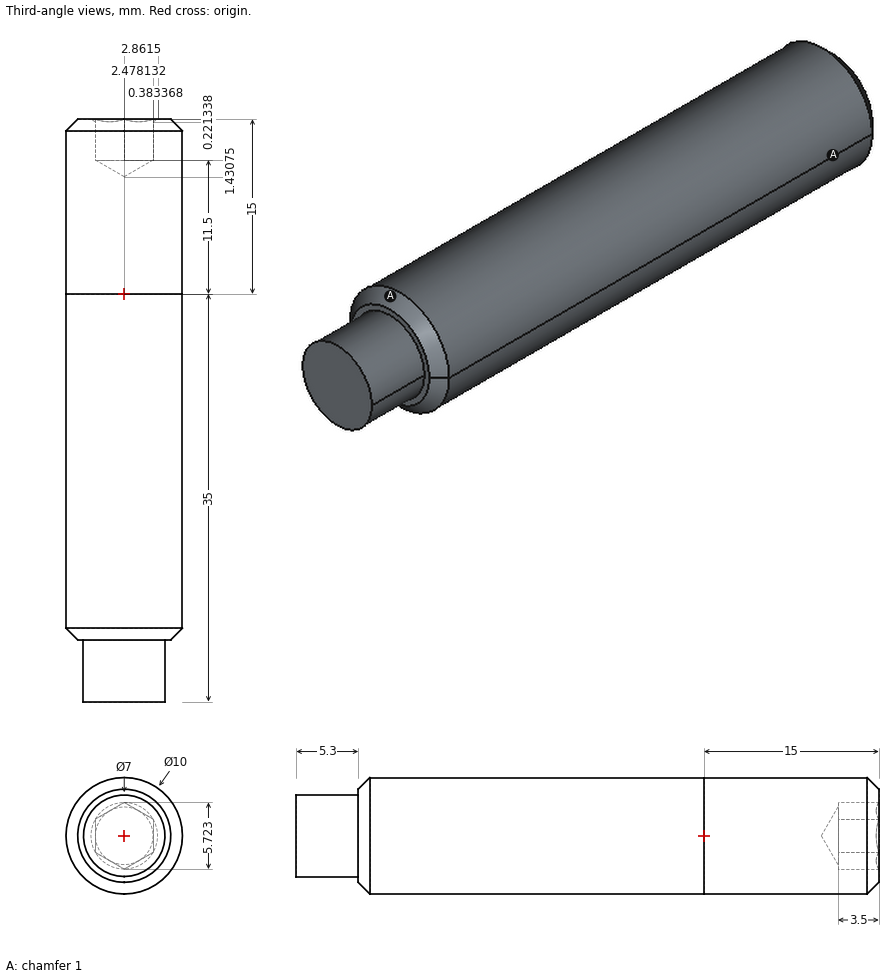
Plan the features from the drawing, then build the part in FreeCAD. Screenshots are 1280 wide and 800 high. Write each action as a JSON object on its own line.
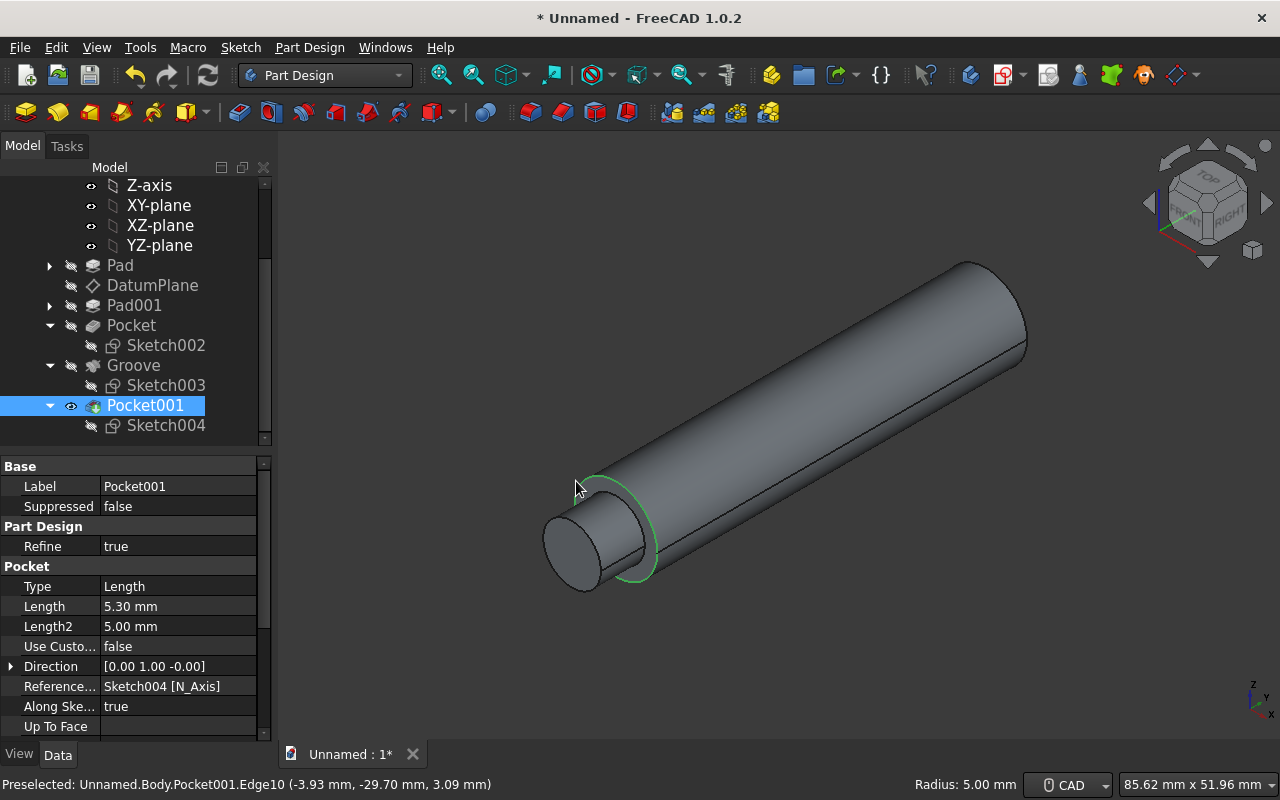
{"action": "key", "text": "2"}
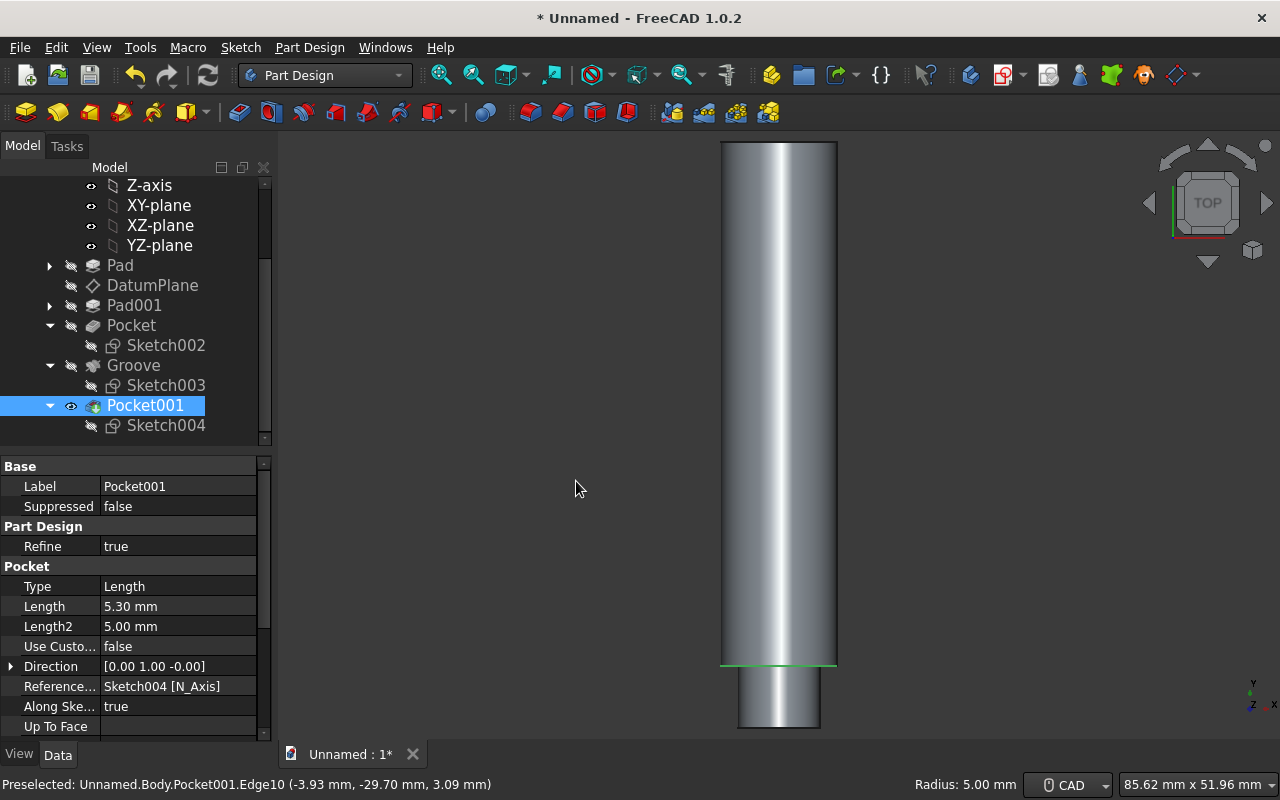
{"action": "key", "text": "0"}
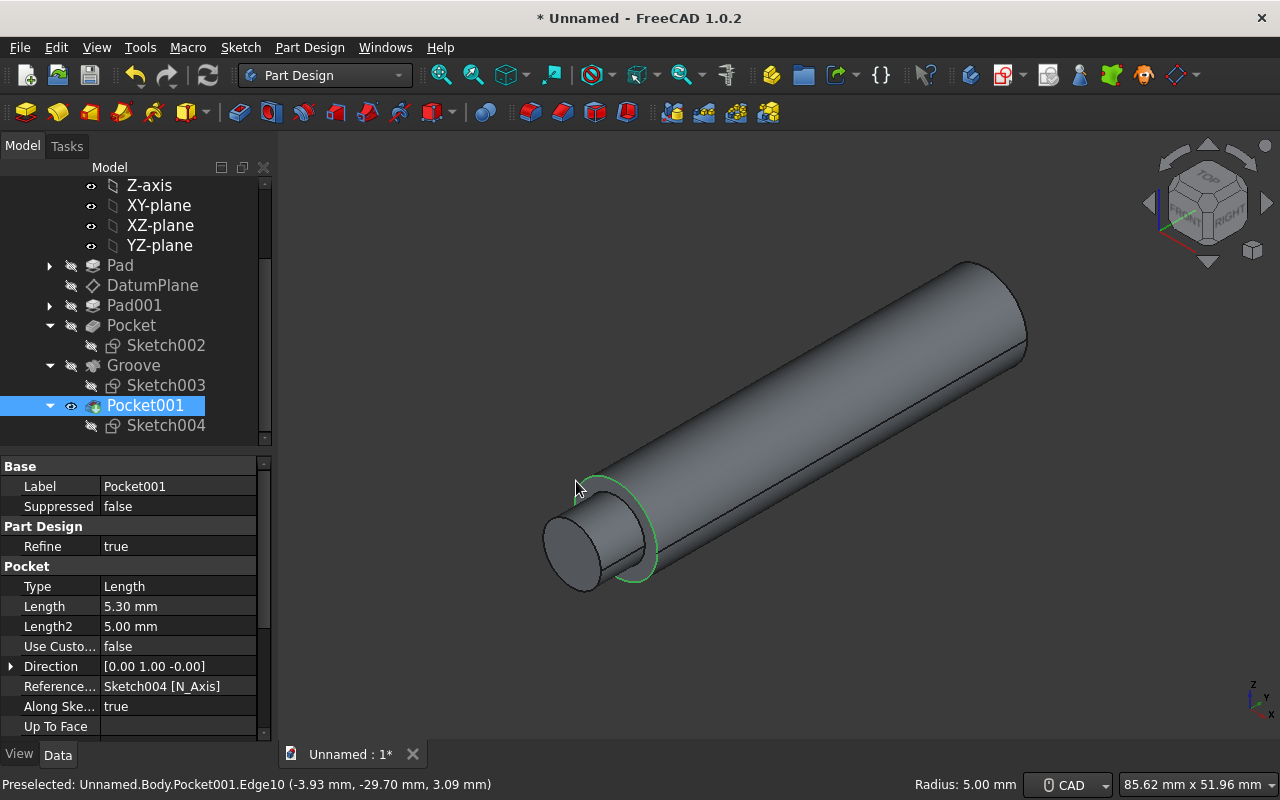
{"action": "key", "text": "1"}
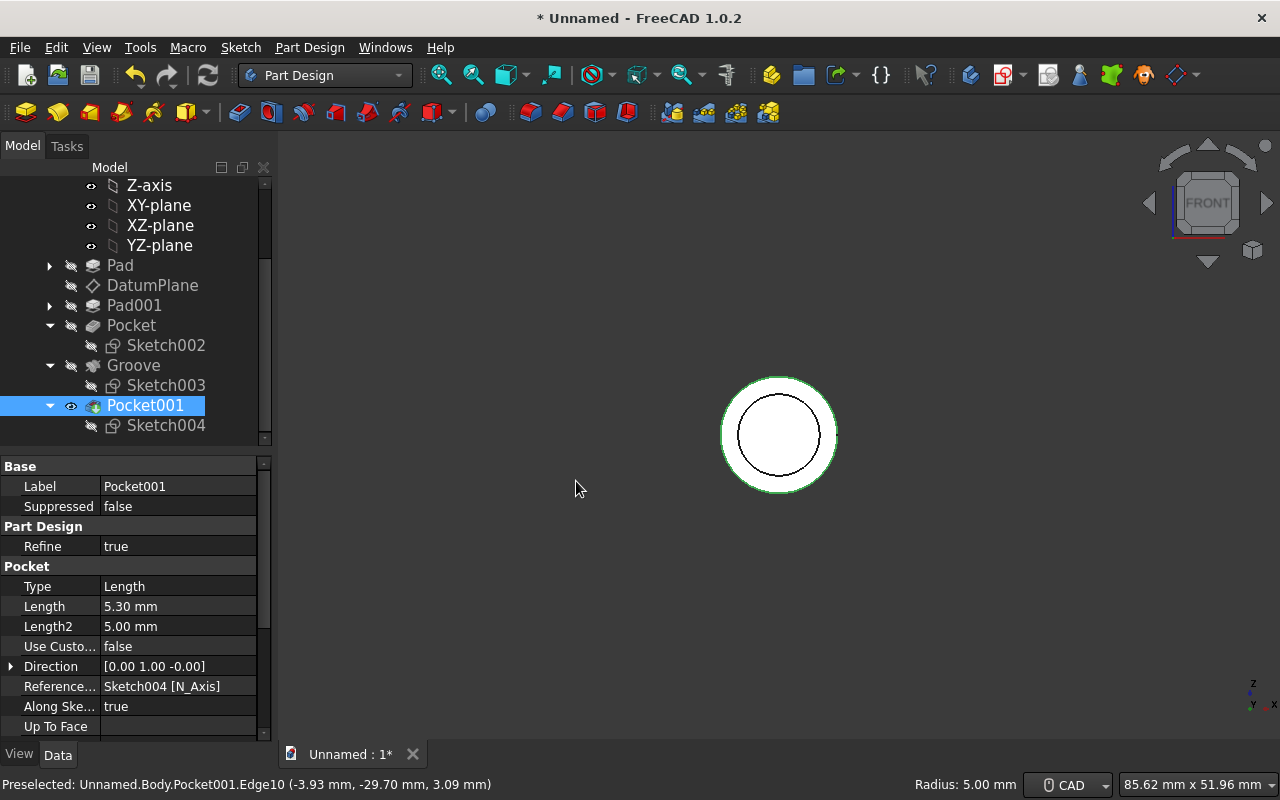
{"action": "left_click", "coordinate": [442, 76]}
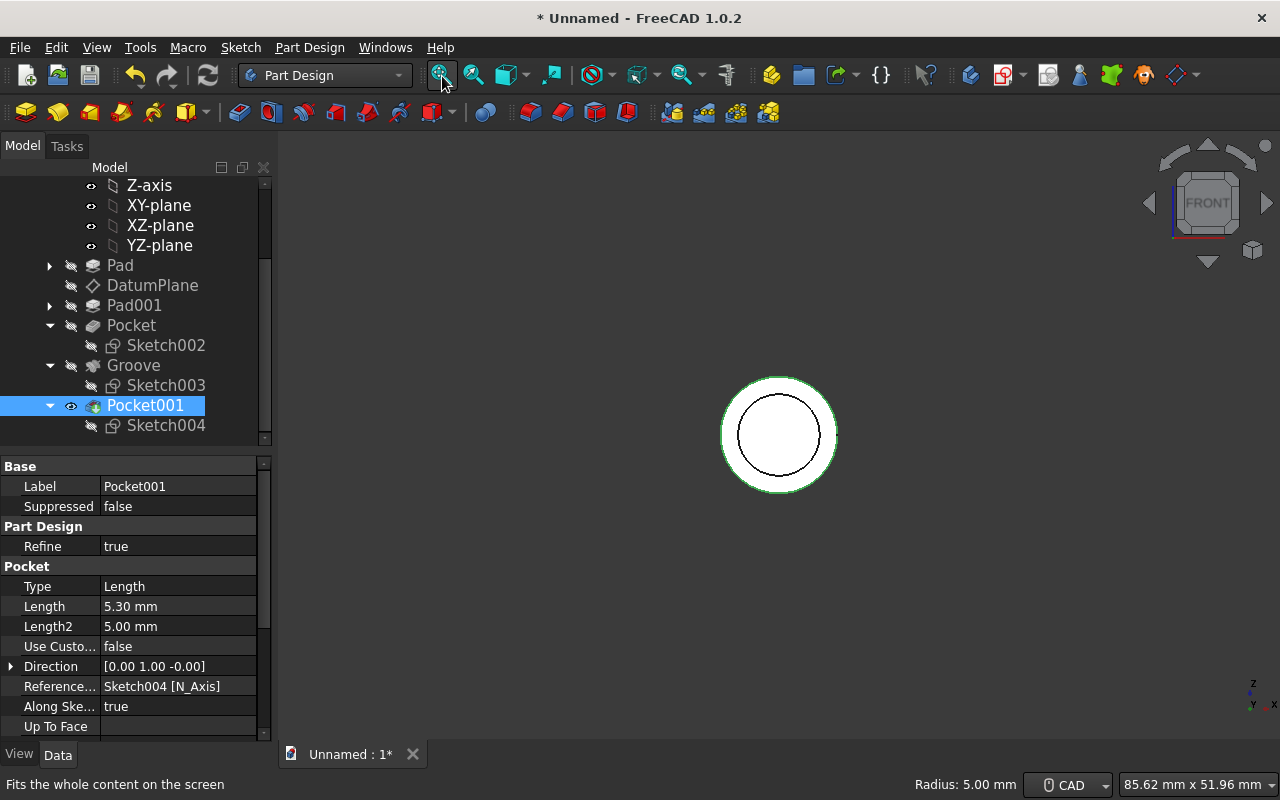
{"action": "key", "text": "3"}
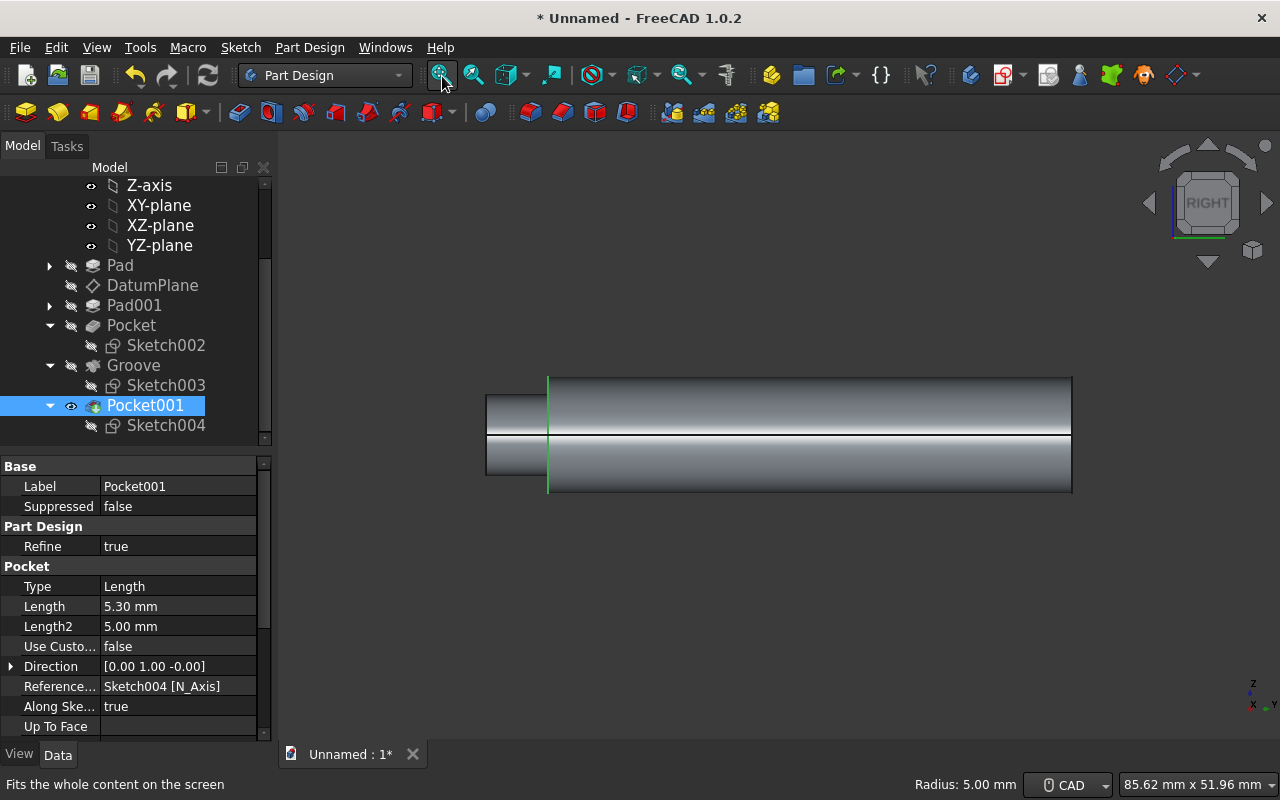
{"action": "left_click", "coordinate": [1072, 400], "text": "ctrl"}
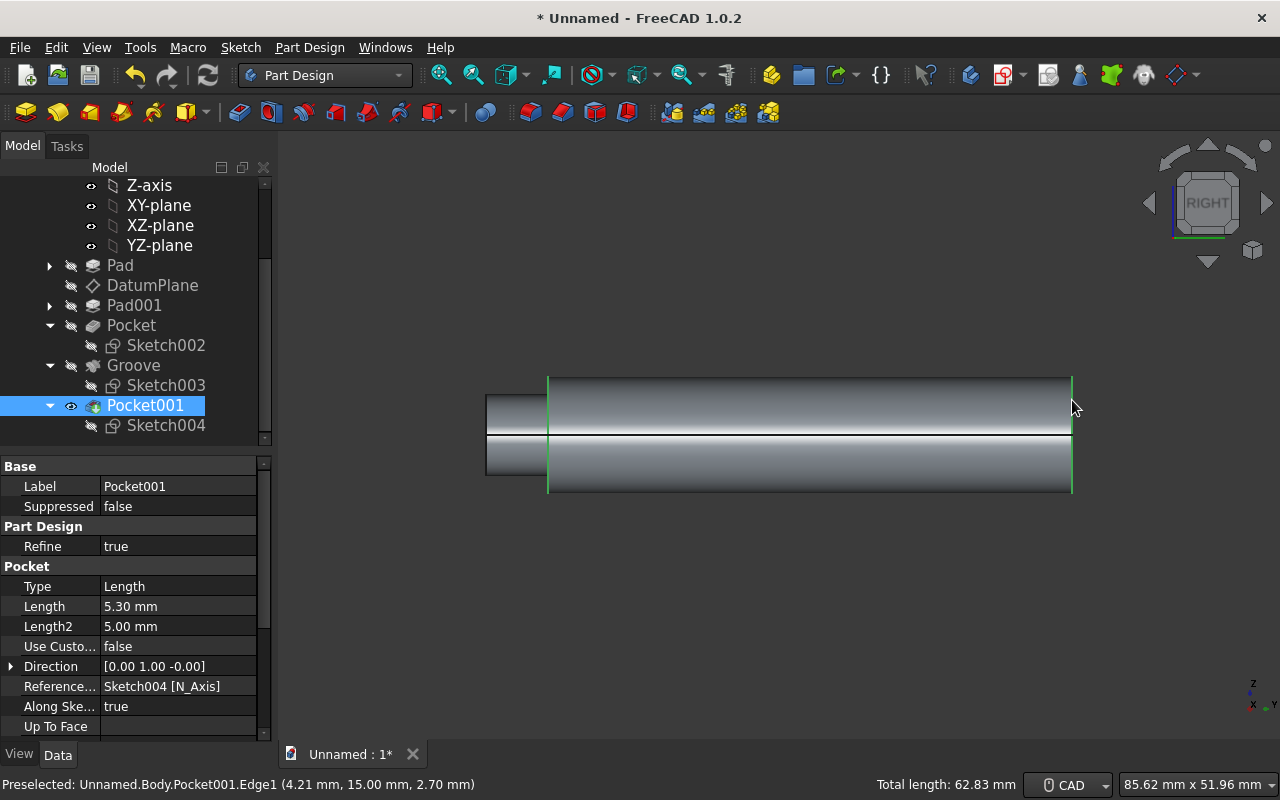
{"action": "left_click", "coordinate": [564, 112]}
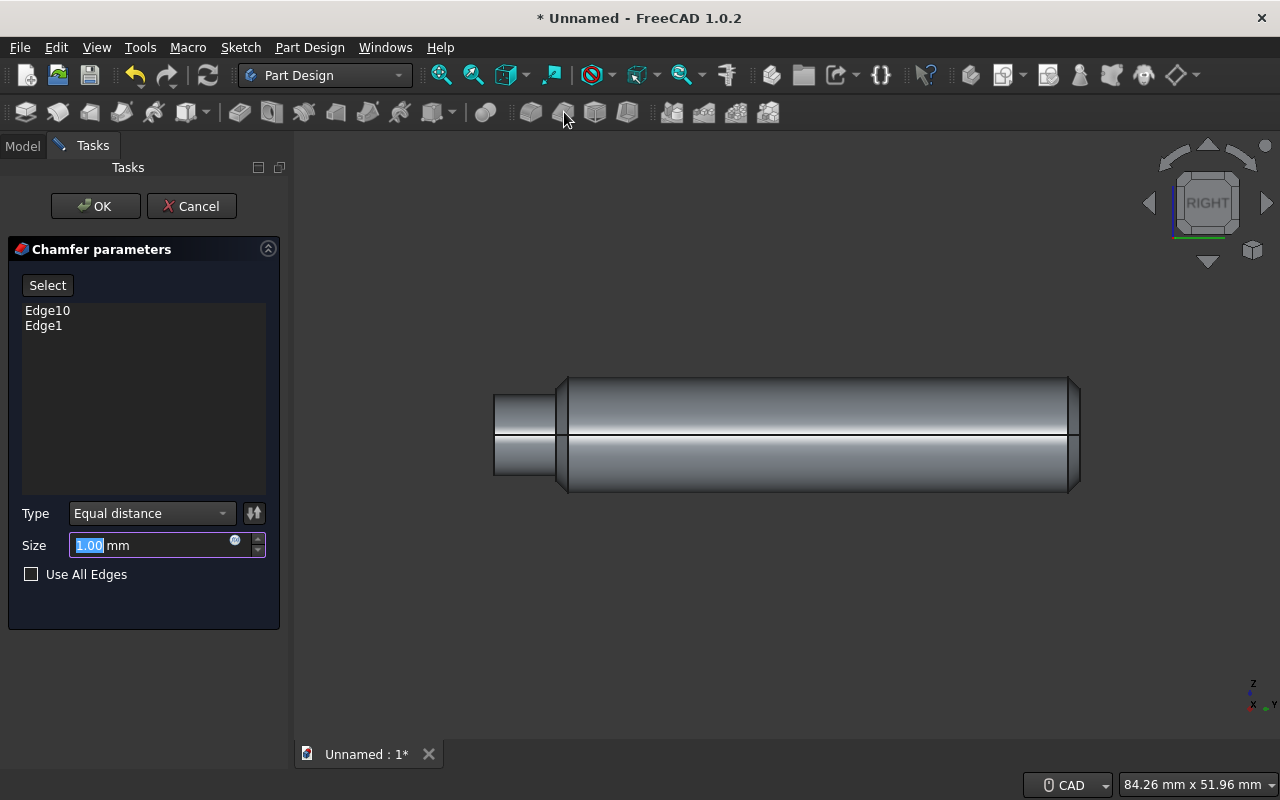
{"action": "type", "text": "1"}
{"action": "key", "text": "Tab"}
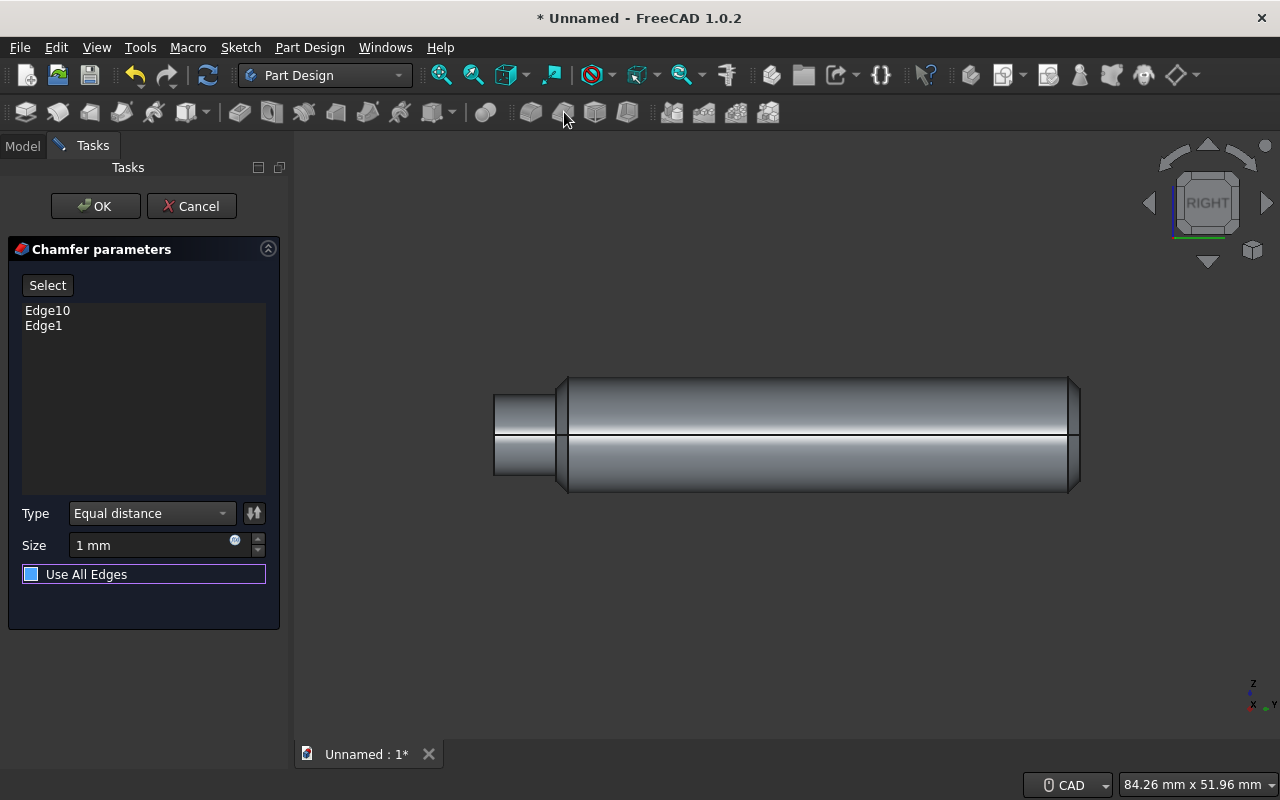
{"action": "left_click", "coordinate": [96, 206]}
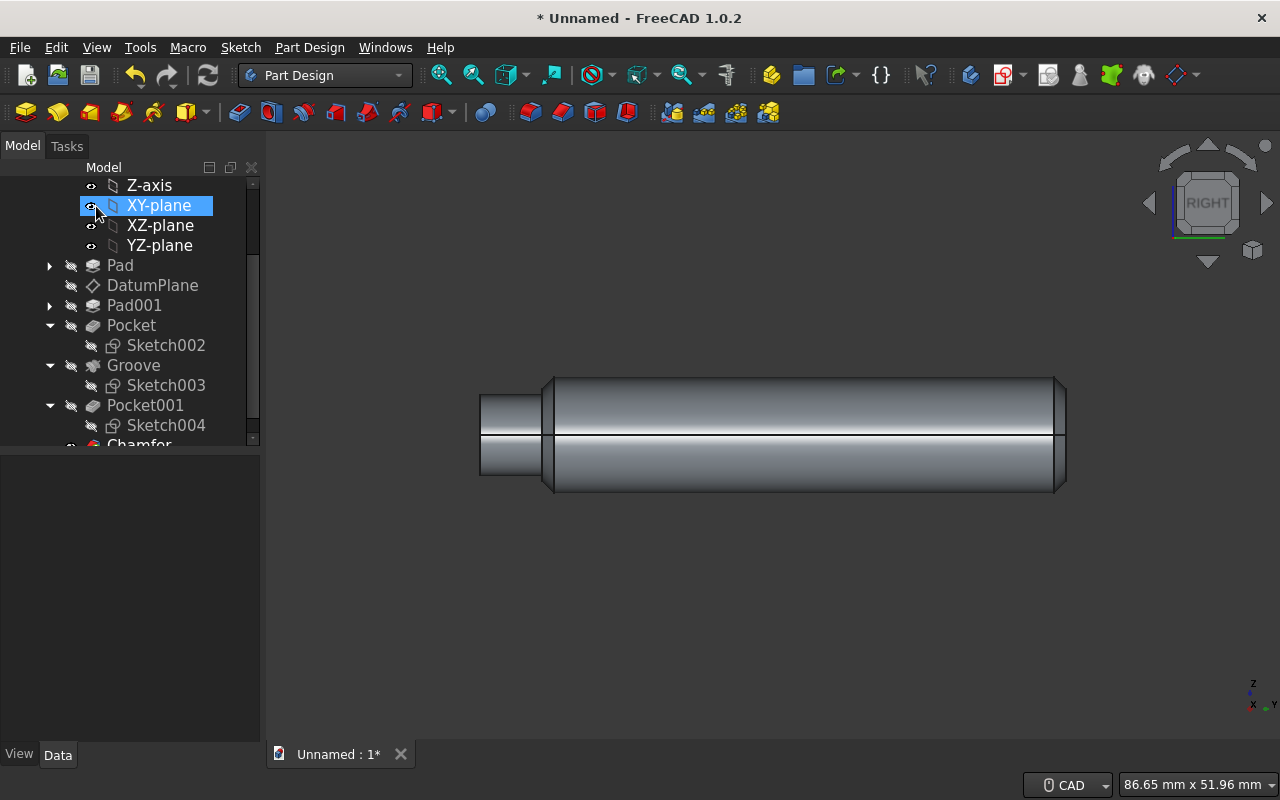
{"action": "key", "text": "0"}